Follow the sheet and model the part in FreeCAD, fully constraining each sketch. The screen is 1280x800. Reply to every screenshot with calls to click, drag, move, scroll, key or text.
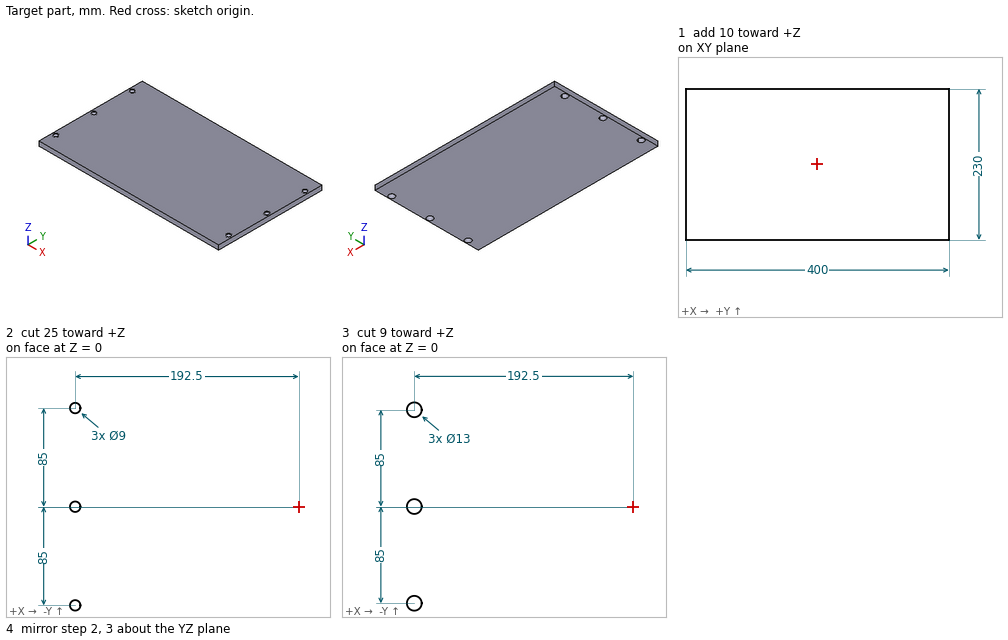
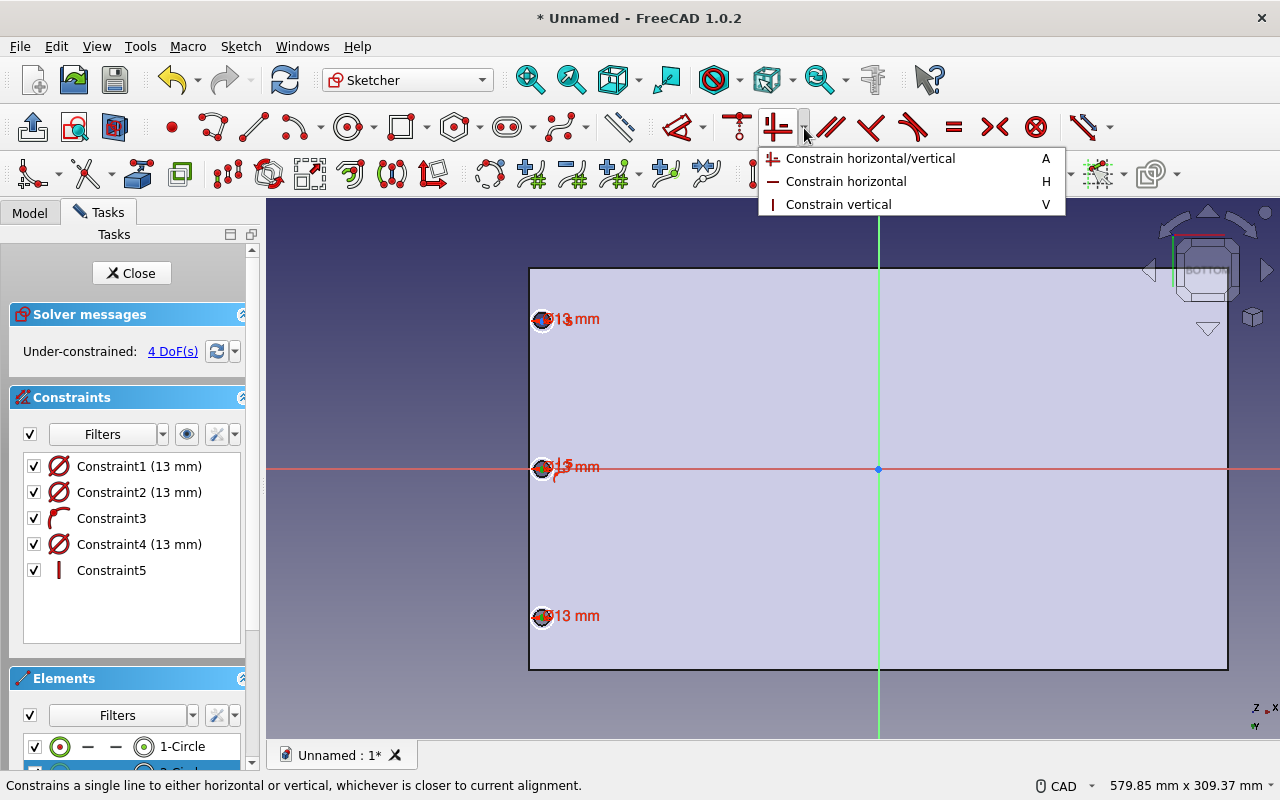
click(912, 204)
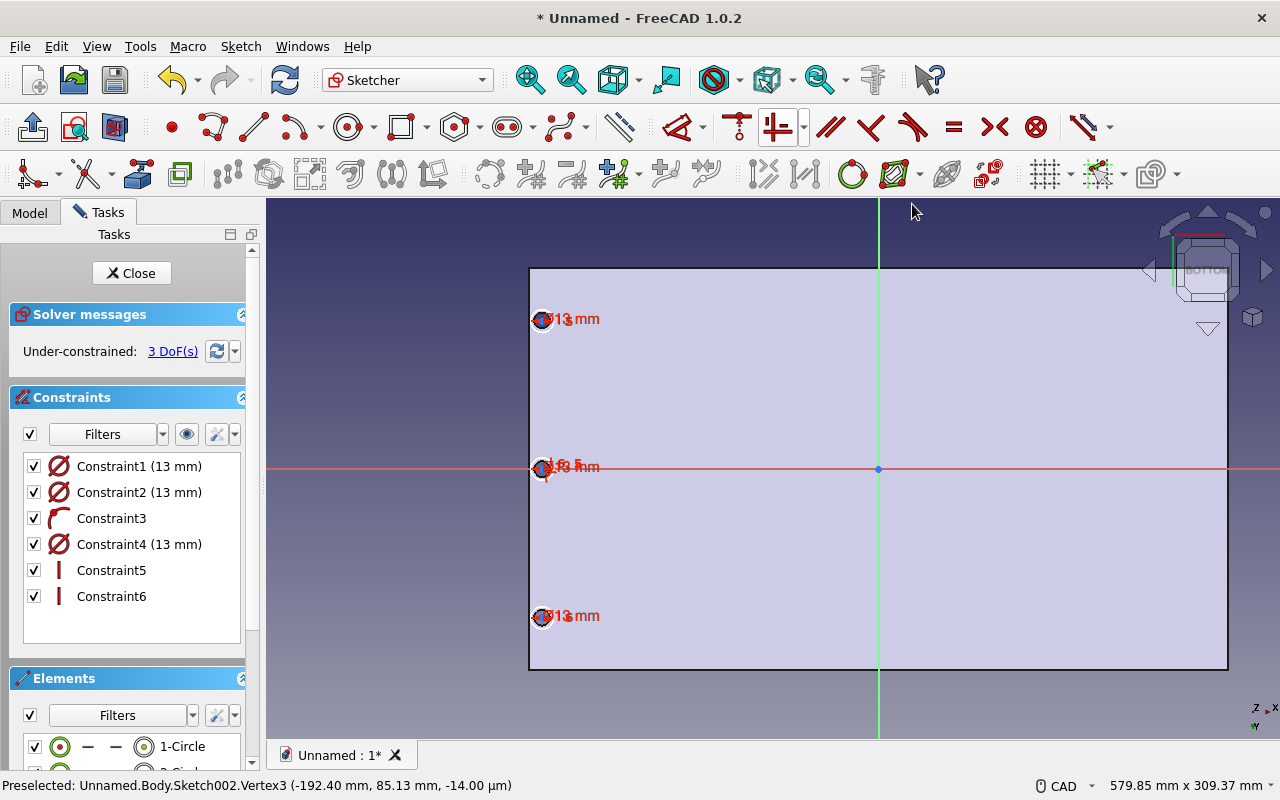
key(d)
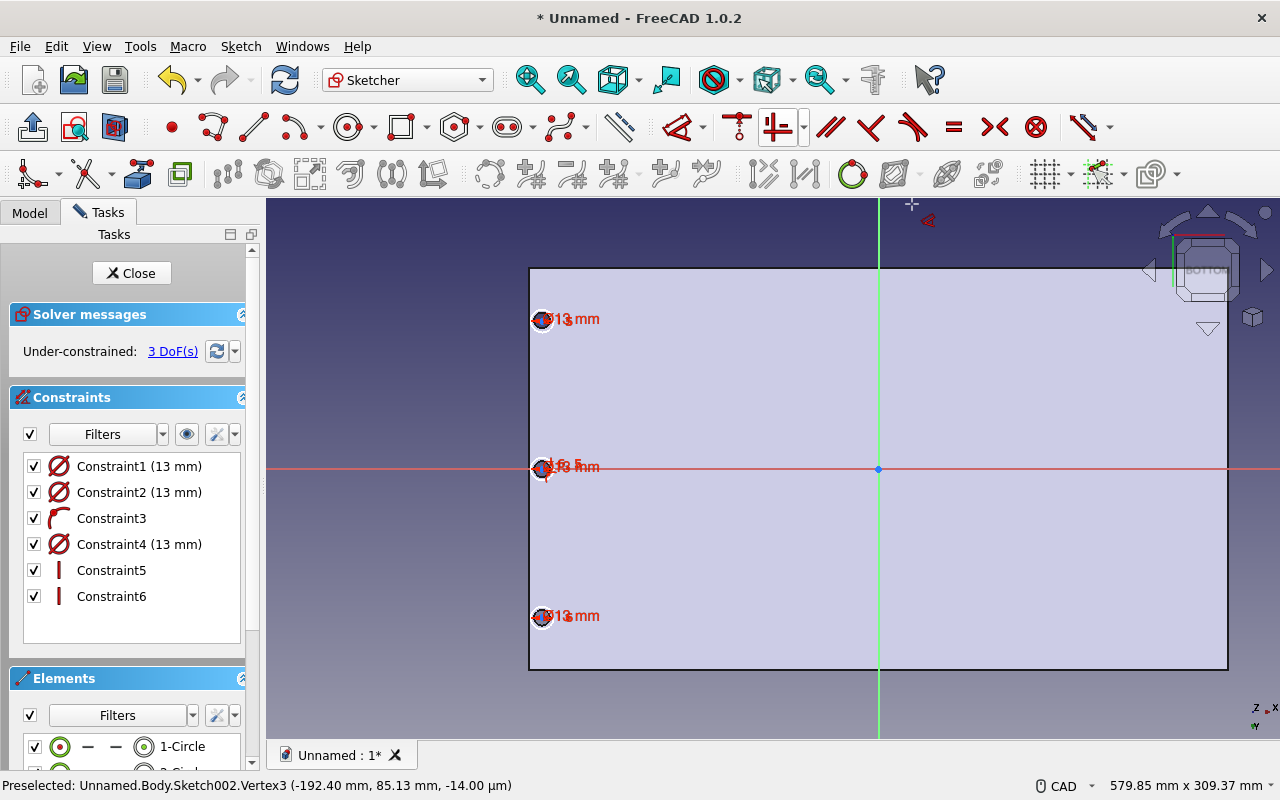
click(542, 321)
click(913, 395)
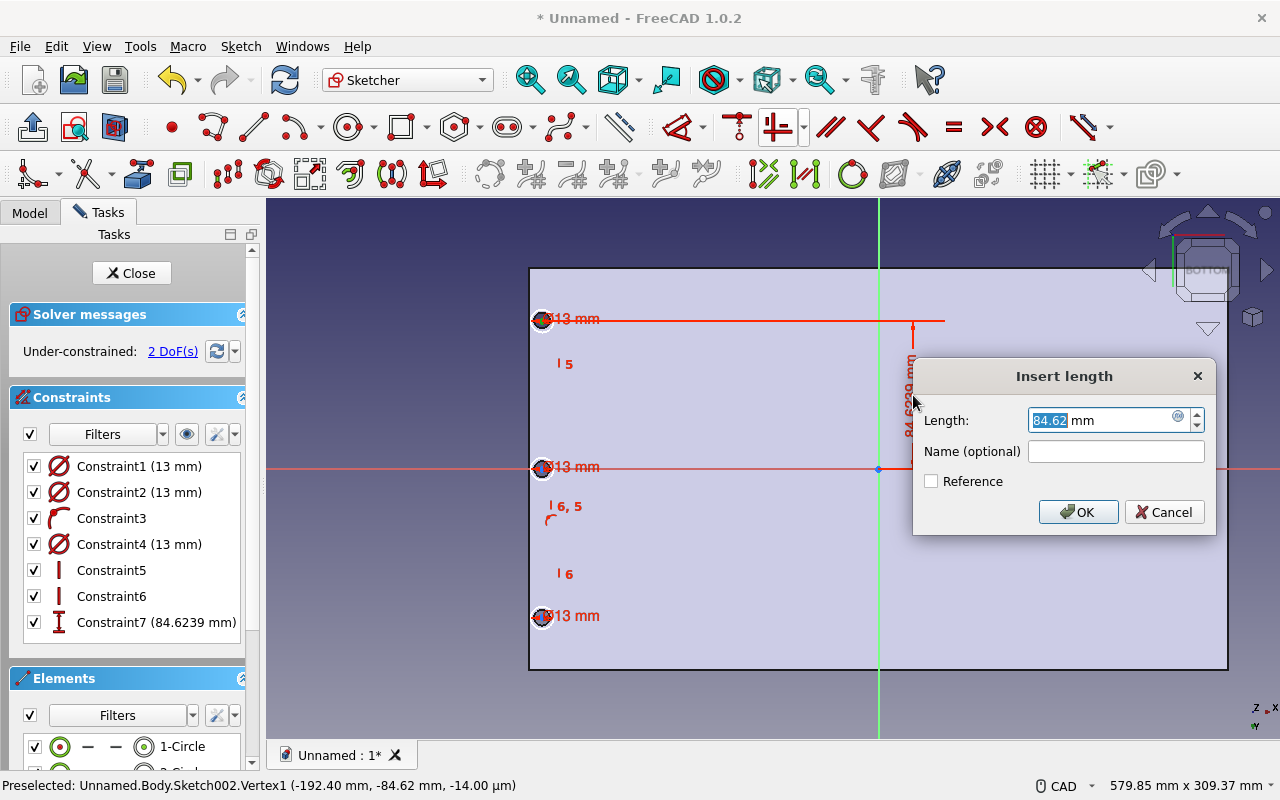
text(85)
key(Return)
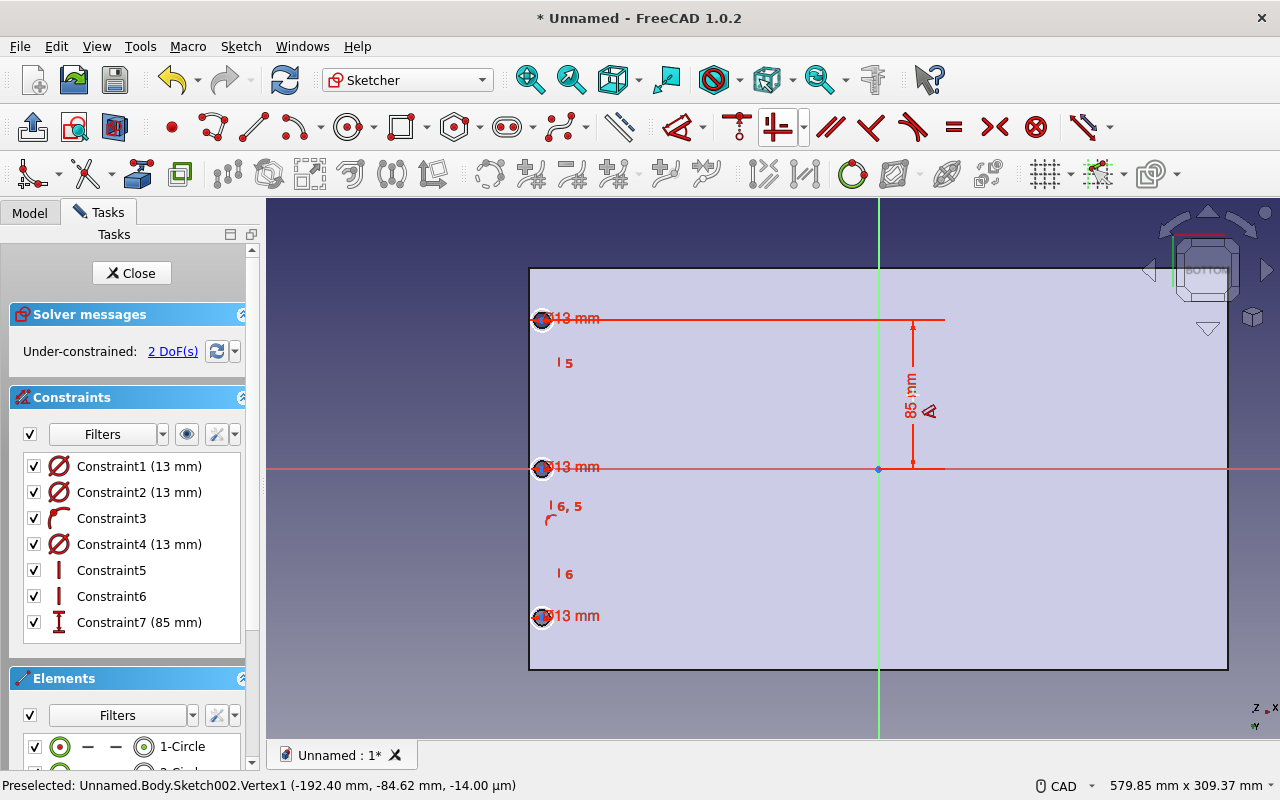
click(542, 618)
click(913, 544)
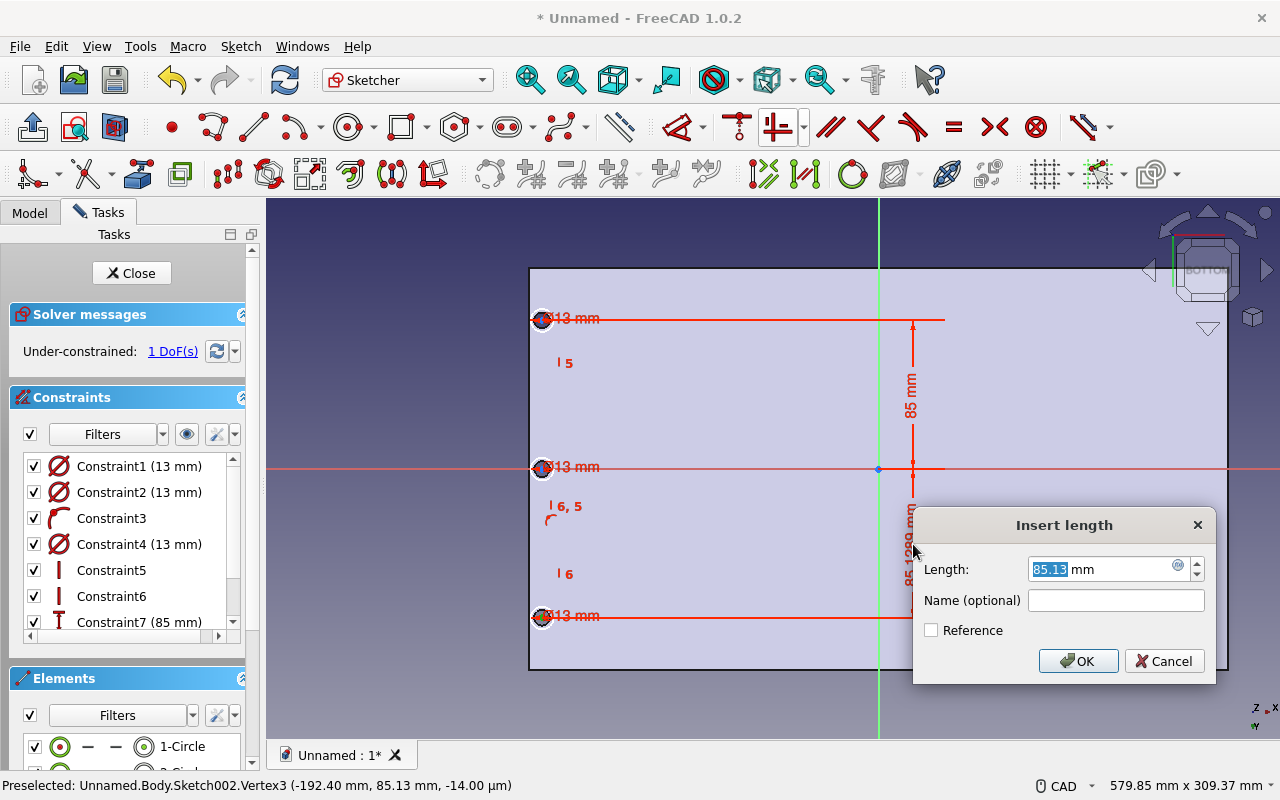
text(85)
key(Return)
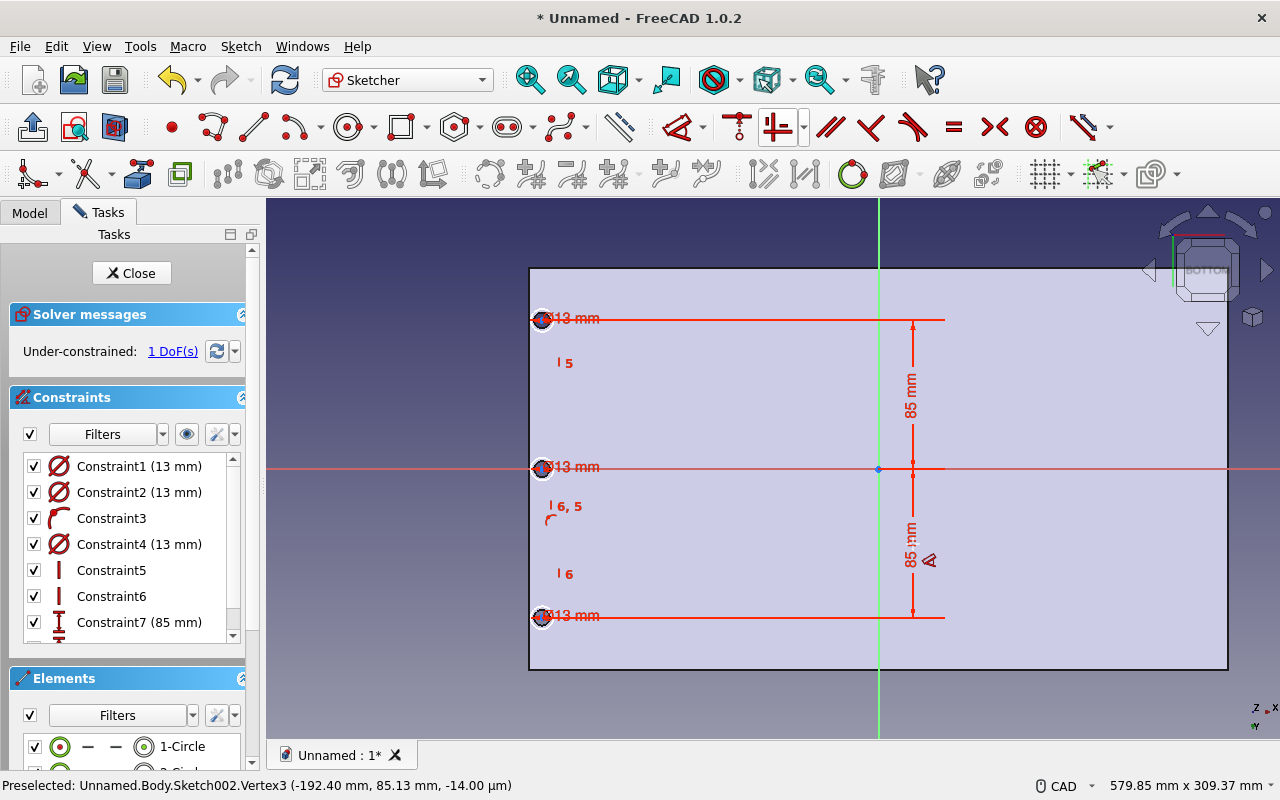
click(542, 320)
click(710, 286)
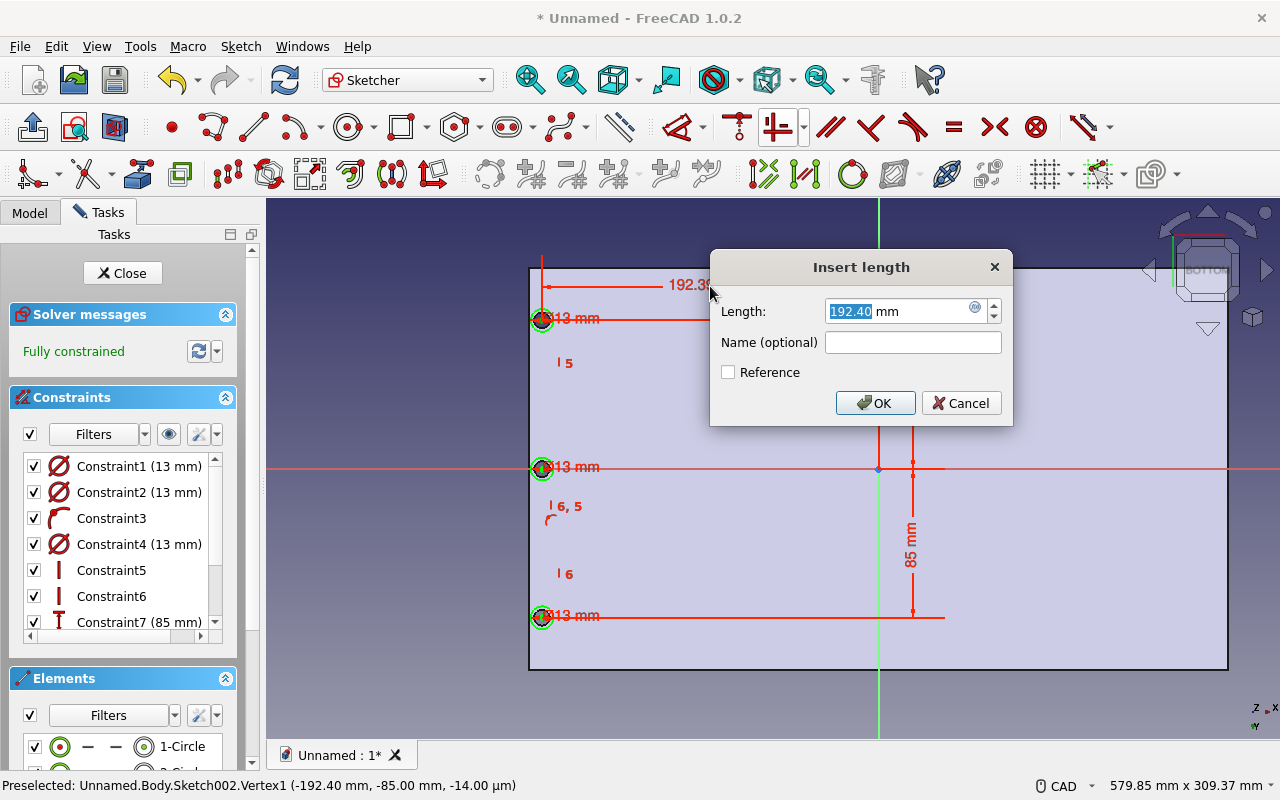
text(192.5)
key(Return)
key(Escape)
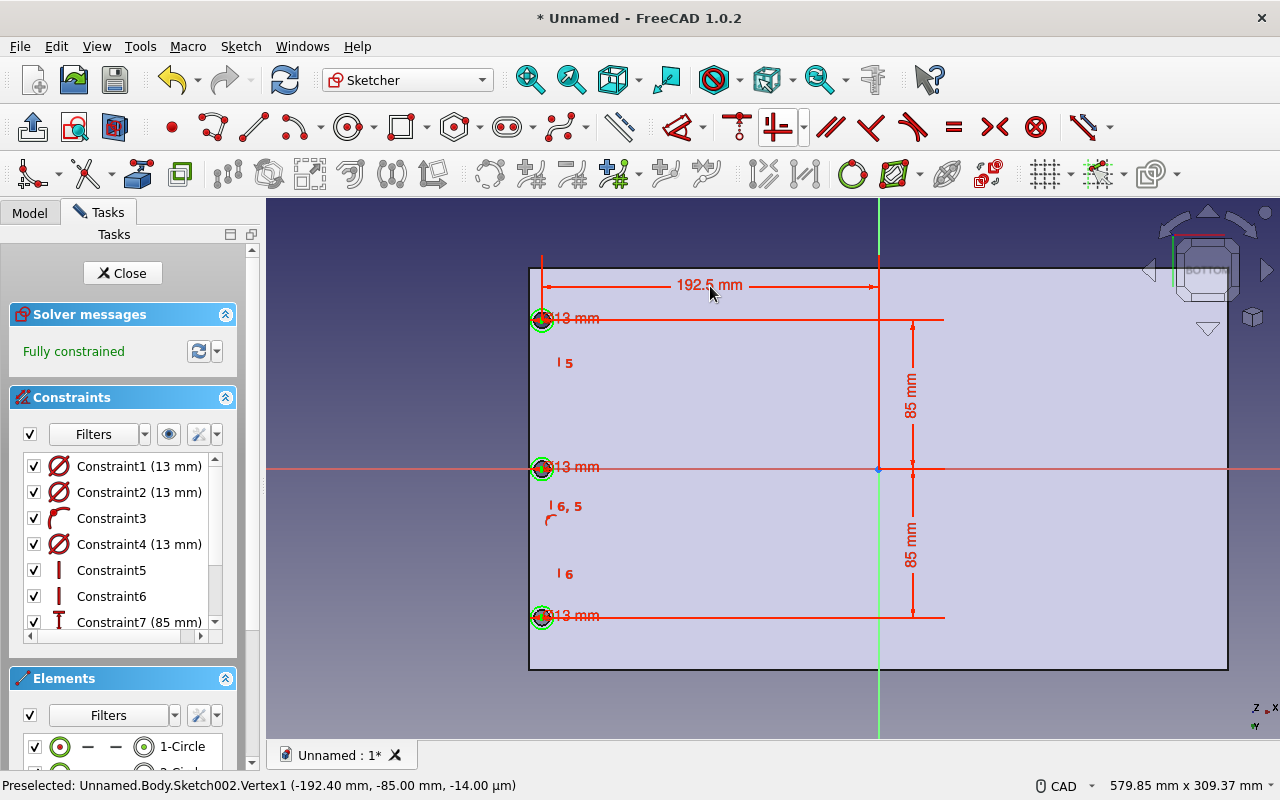
click(123, 273)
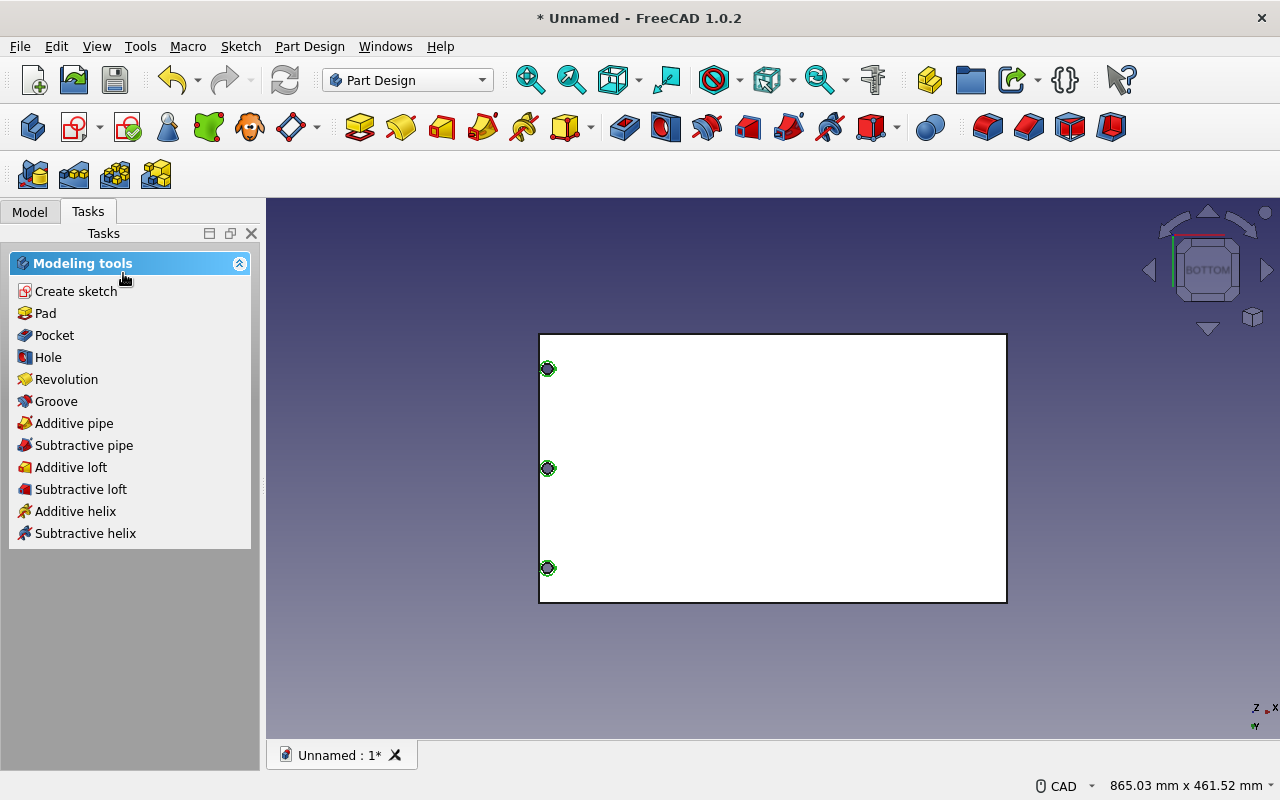
click(625, 128)